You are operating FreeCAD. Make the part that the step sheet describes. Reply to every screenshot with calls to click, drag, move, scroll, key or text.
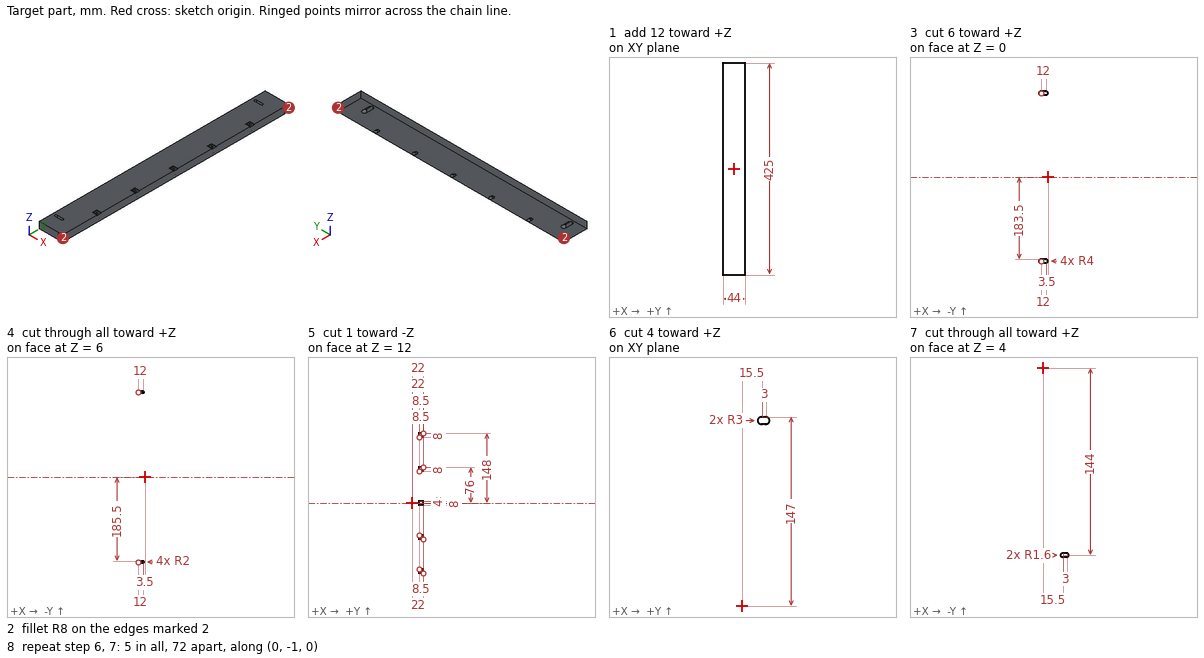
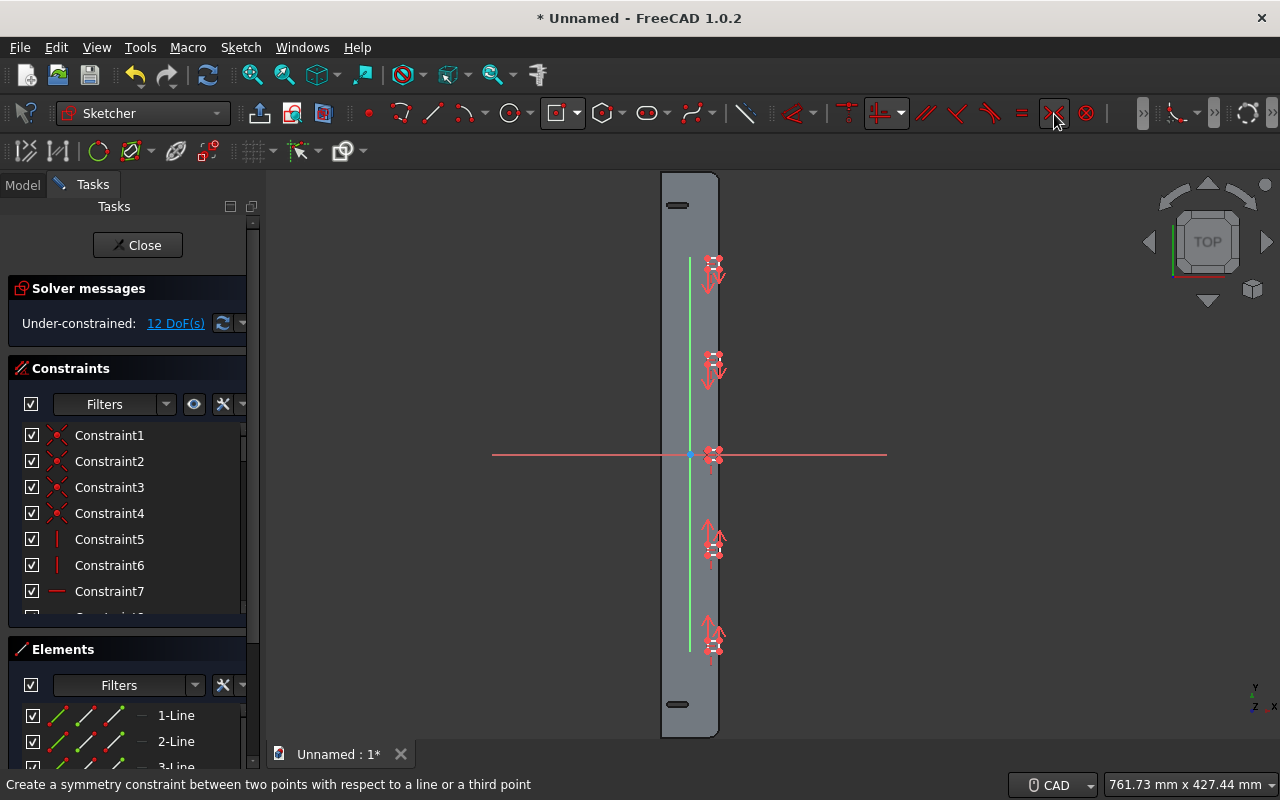
click(792, 114)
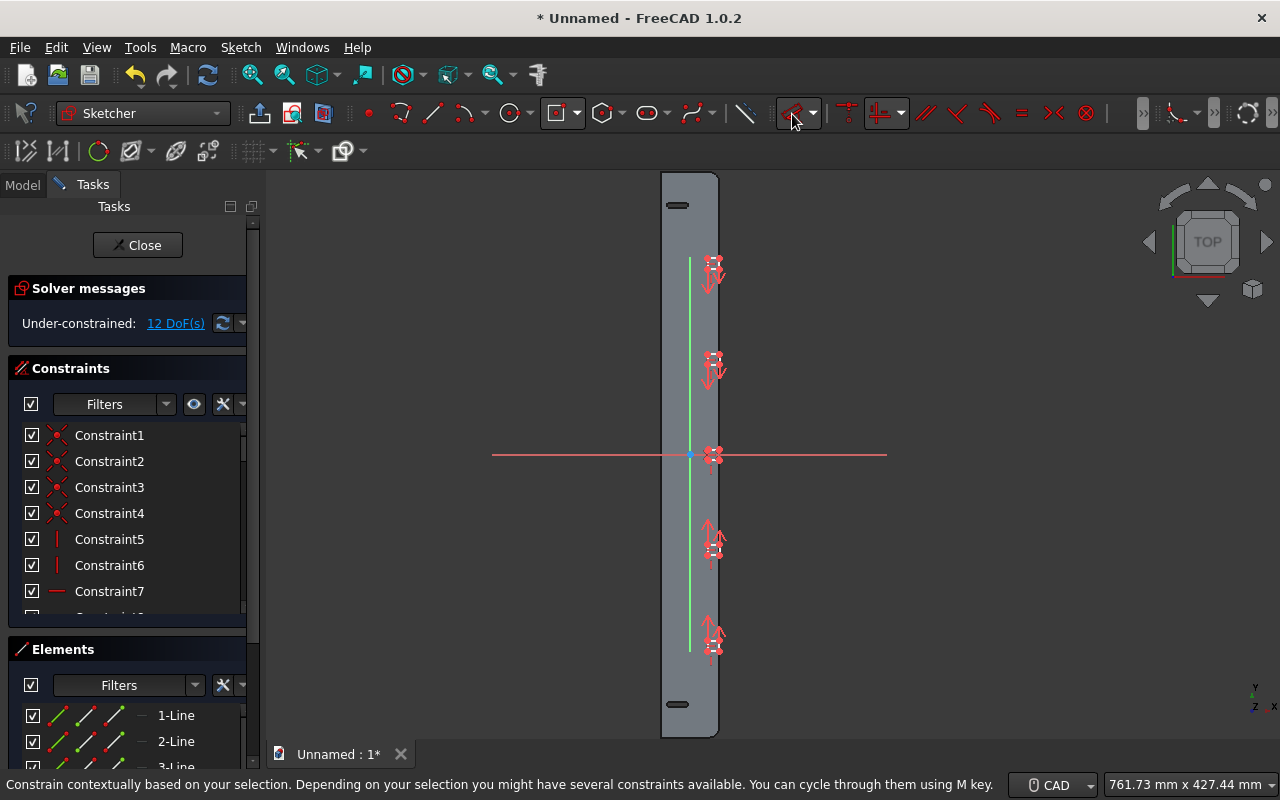
scroll(708, 264, up, 7)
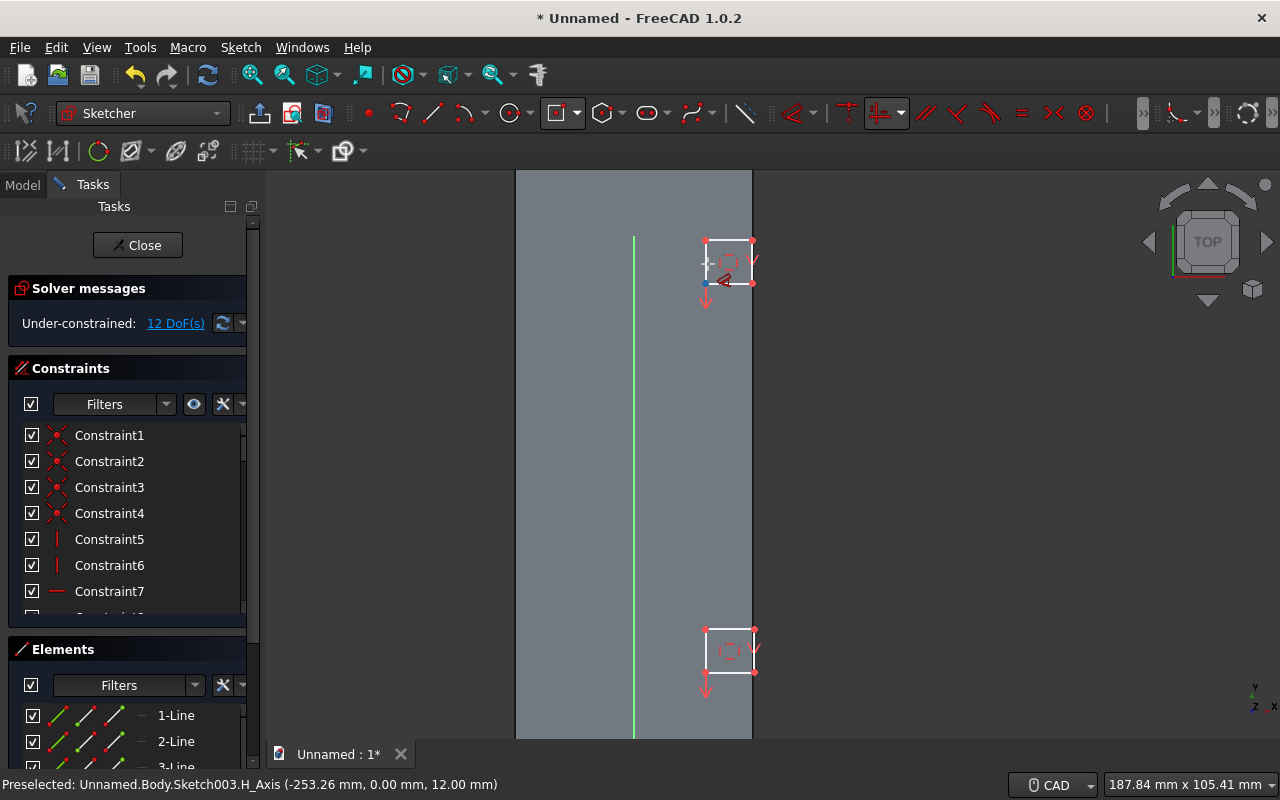
click(706, 262)
click(672, 262)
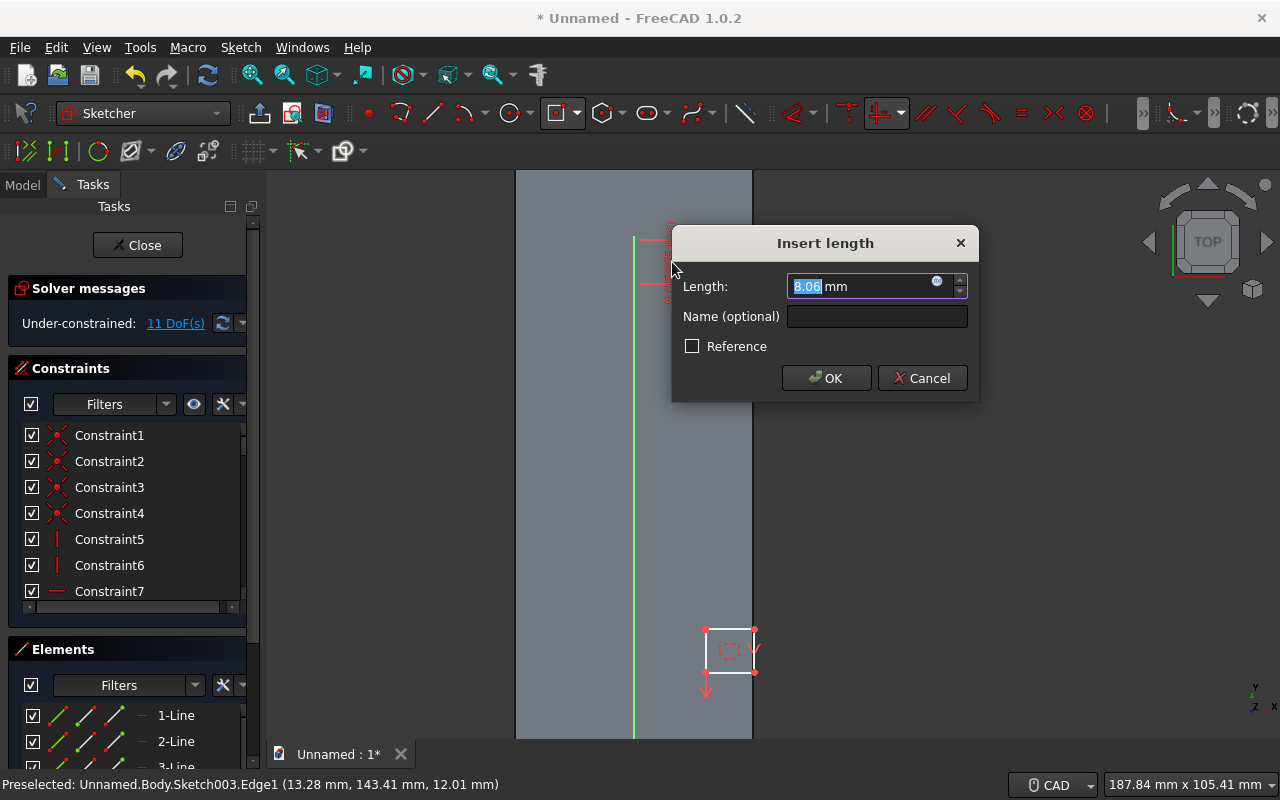
text(8)
key(Return)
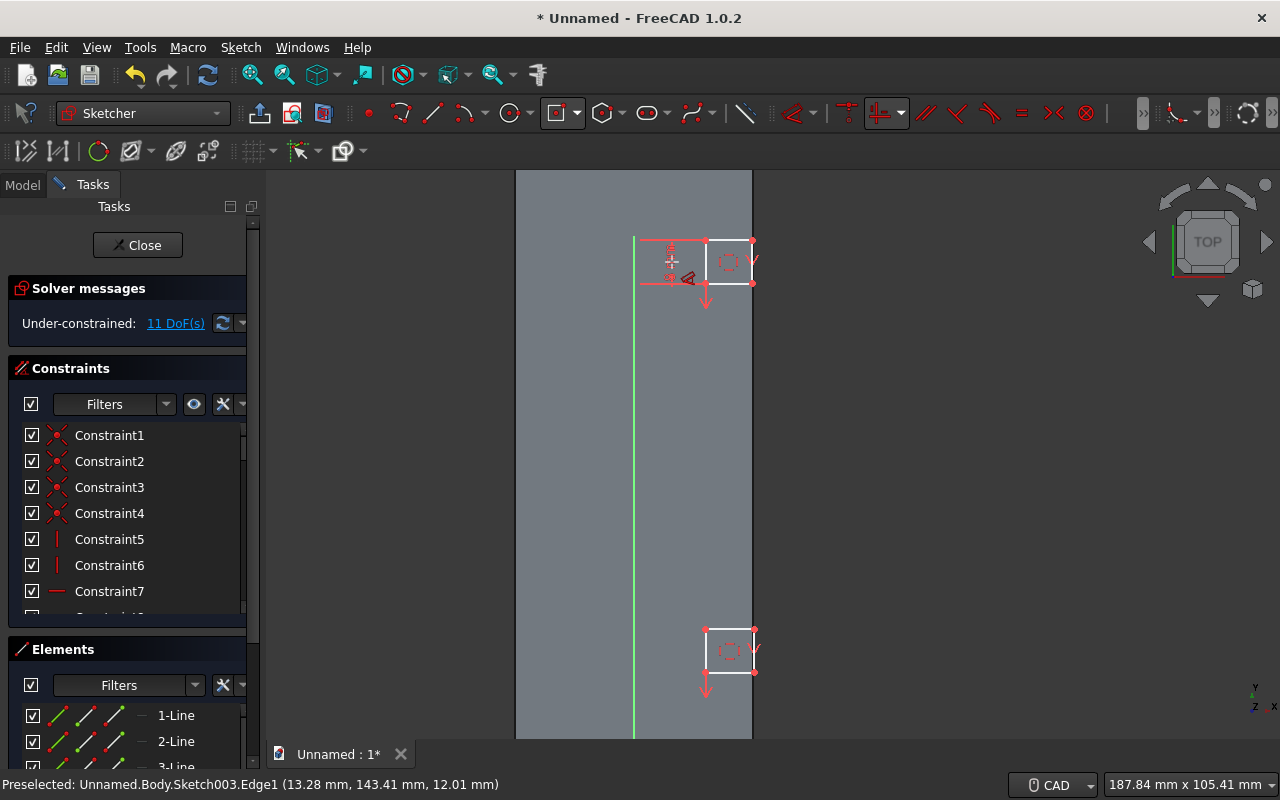
click(706, 642)
click(740, 651)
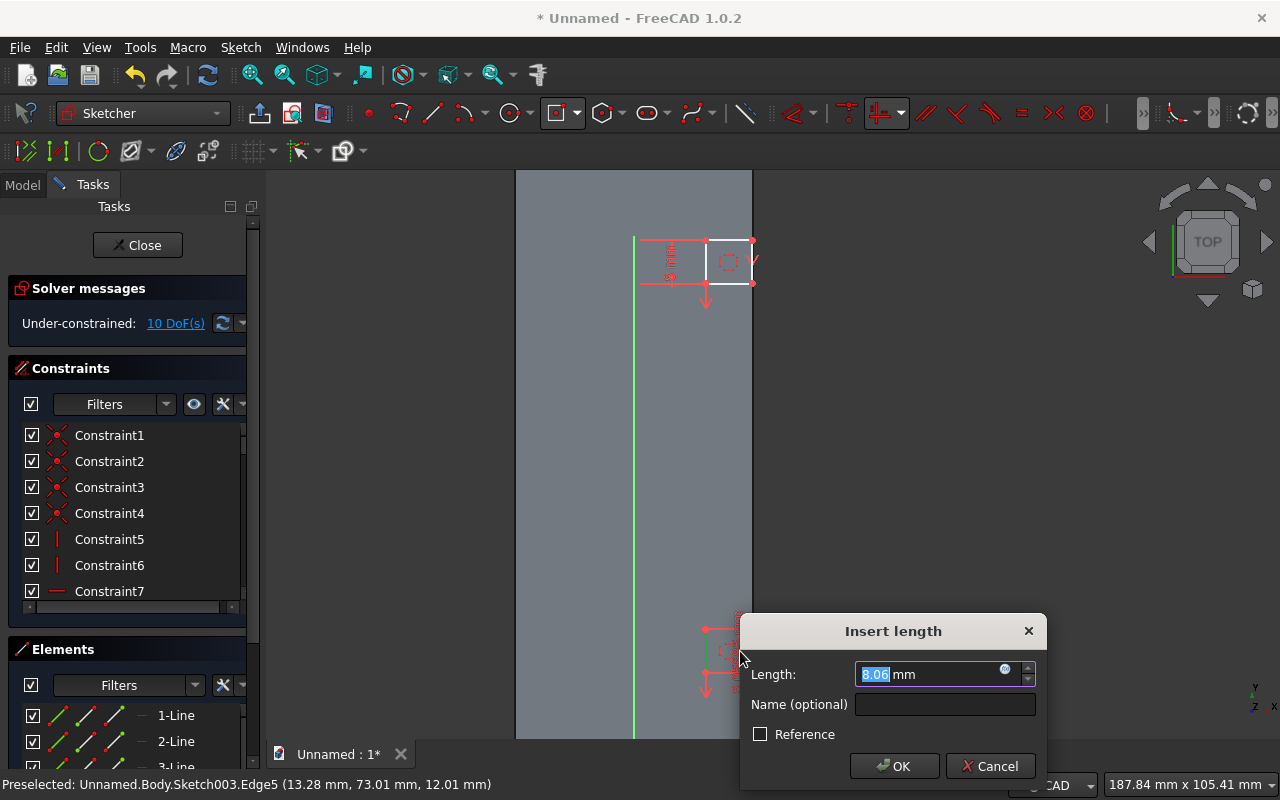
text(8)
key(Return)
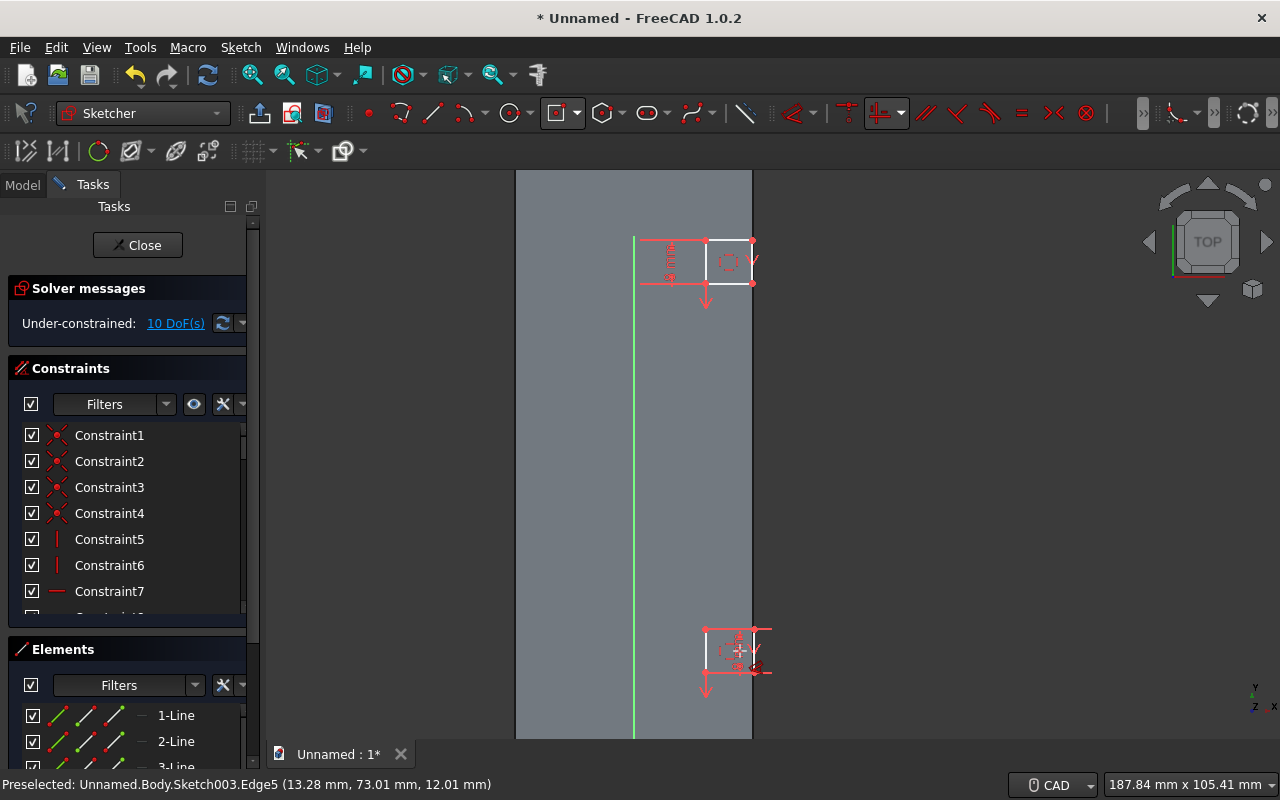
scroll(708, 264, down, 7)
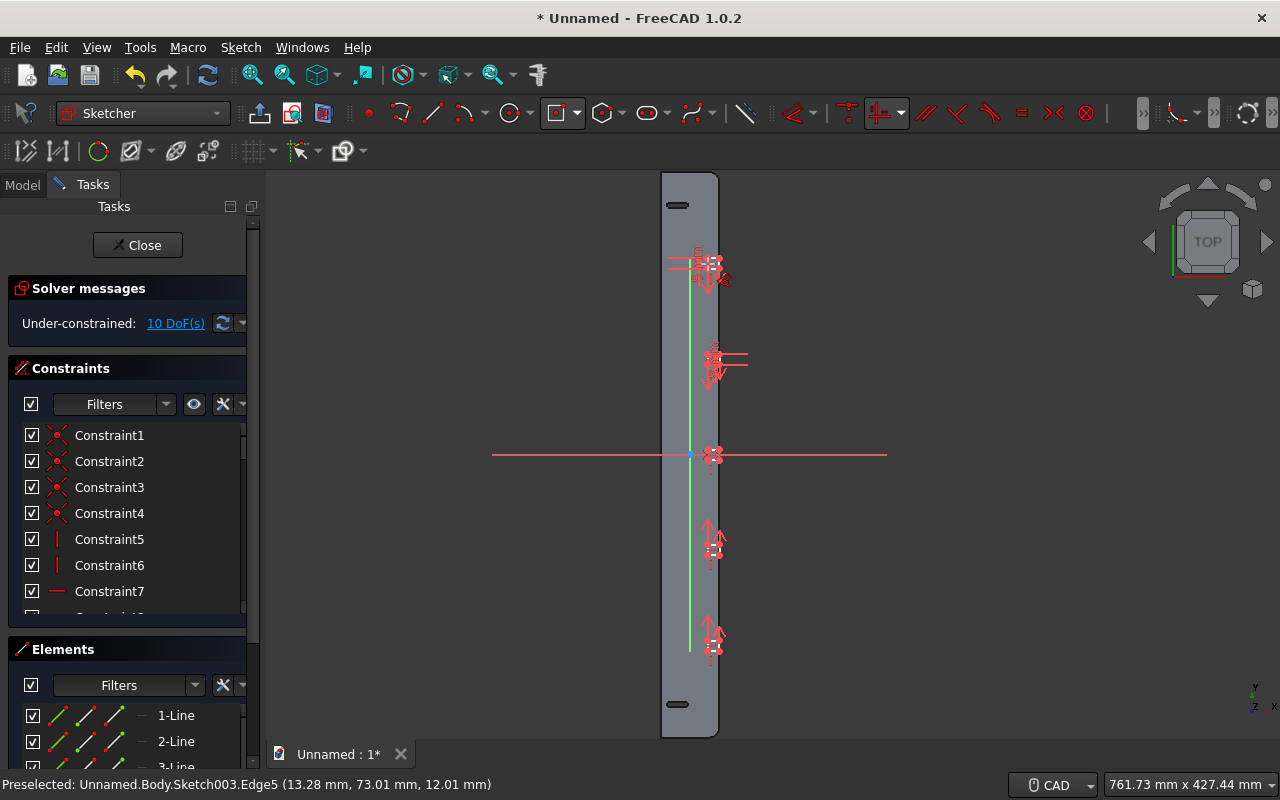
scroll(708, 457, up, 9)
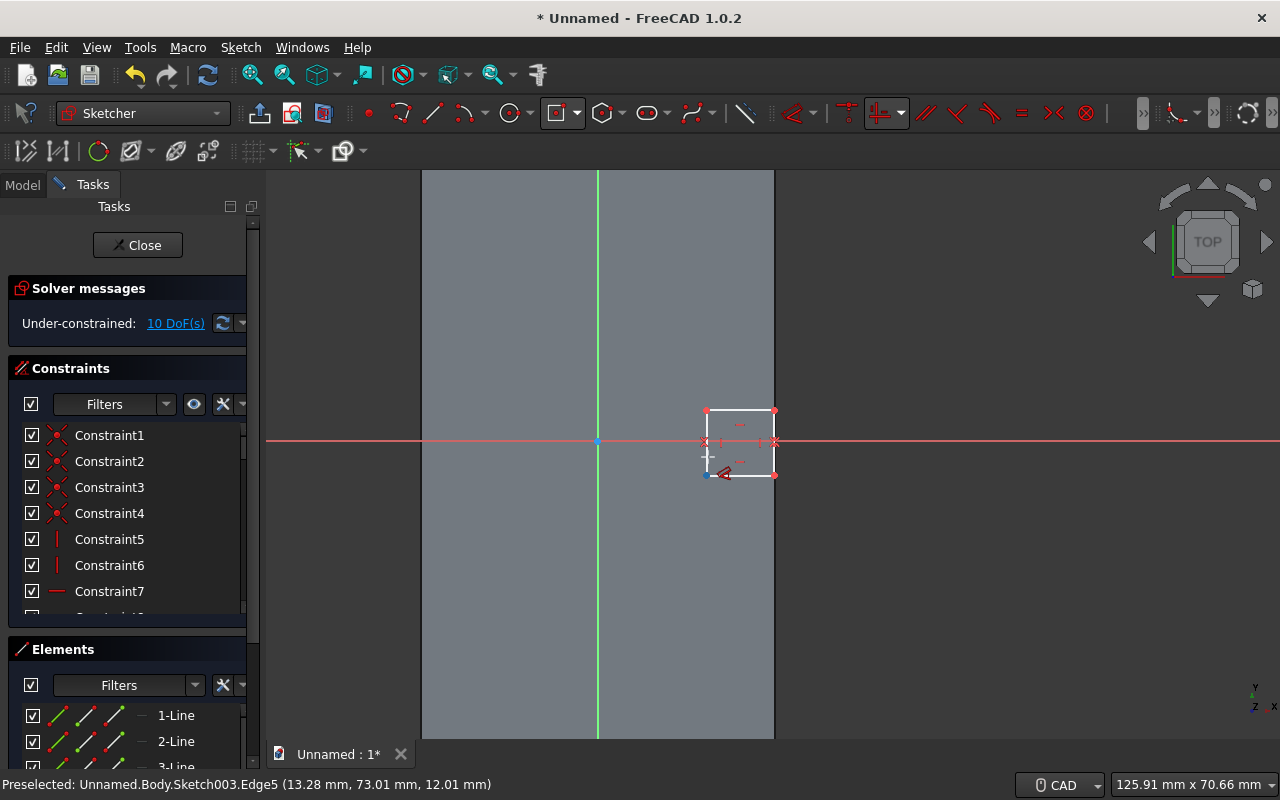
click(707, 456)
click(741, 428)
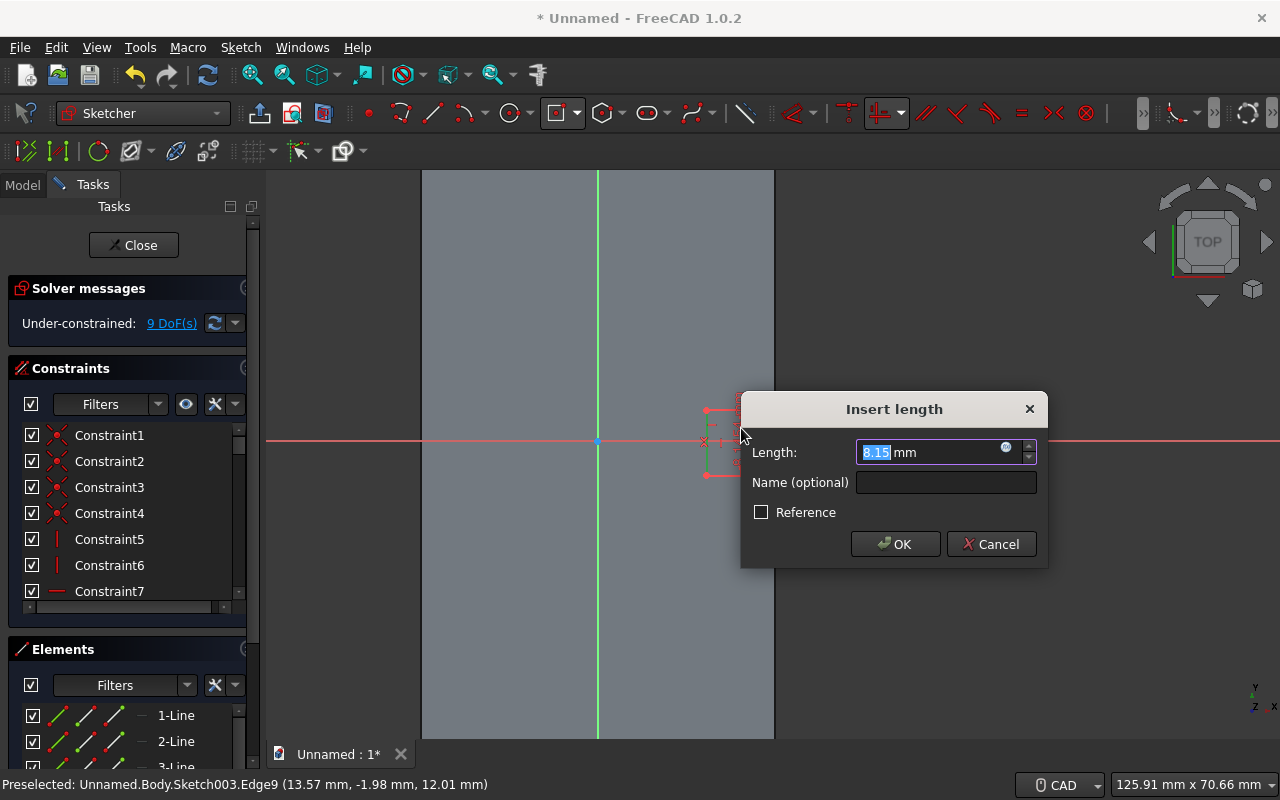
text(8)
key(Return)